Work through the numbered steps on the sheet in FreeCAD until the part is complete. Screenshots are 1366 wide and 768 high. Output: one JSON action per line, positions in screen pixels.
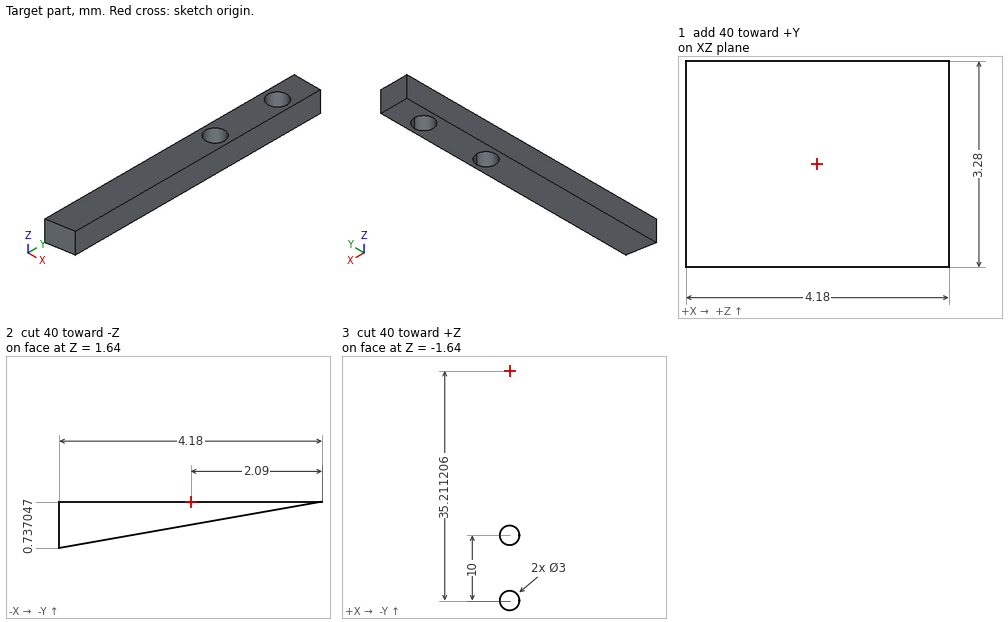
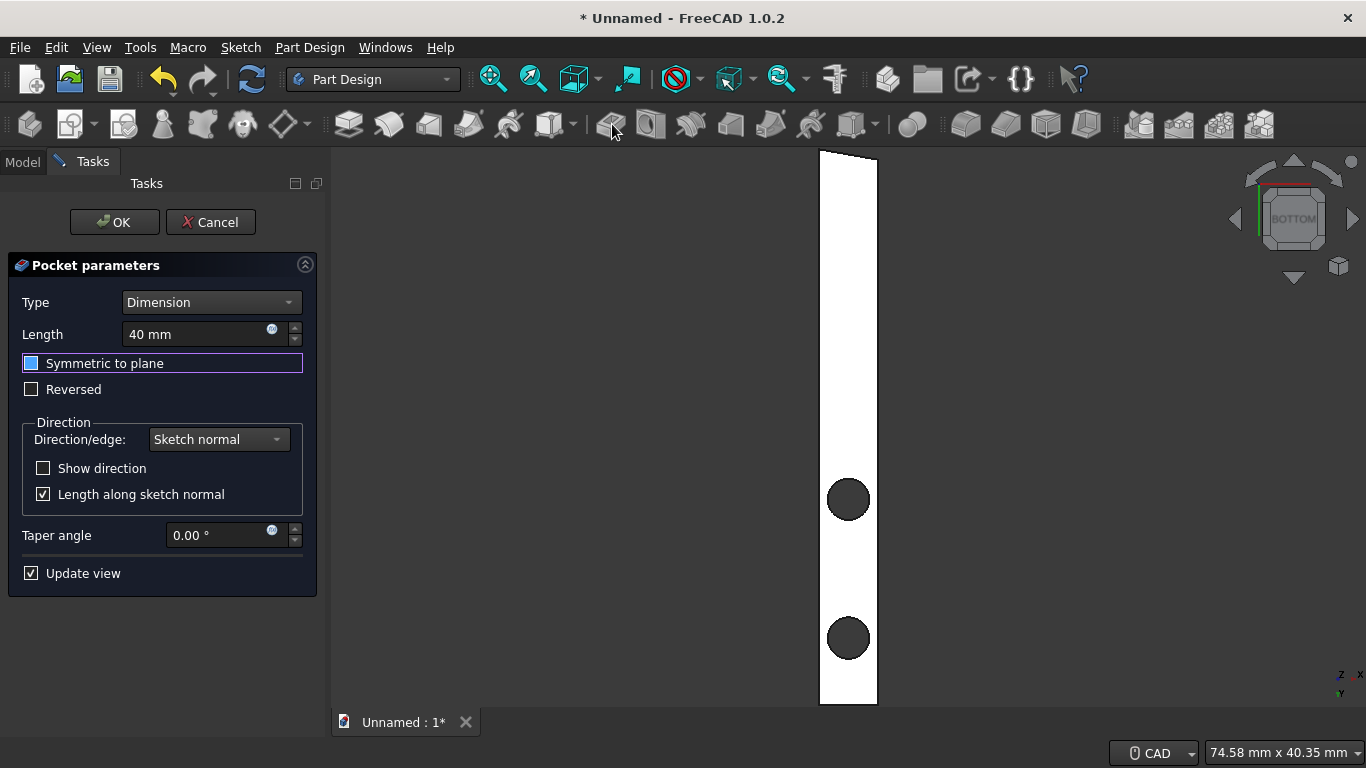
{"action": "left_click", "coordinate": [115, 222]}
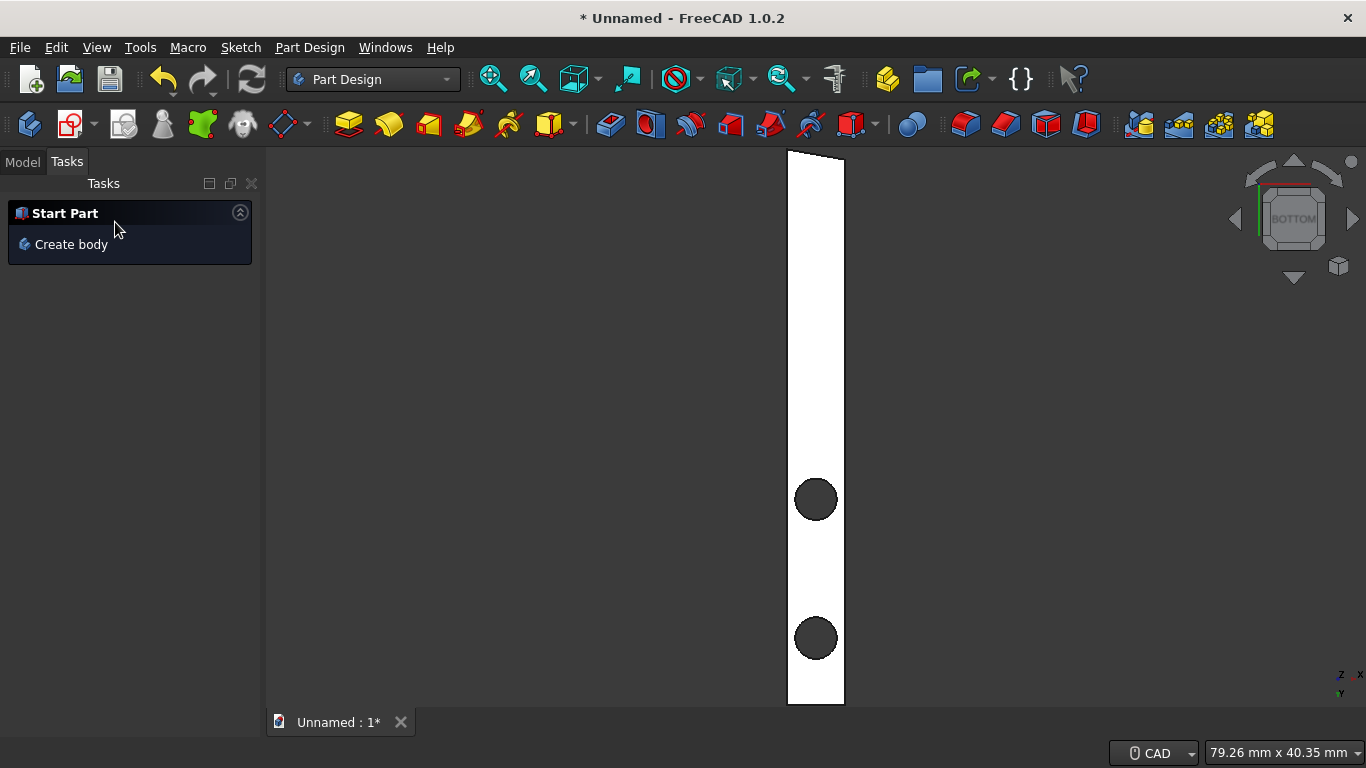
{"action": "key", "text": "0"}